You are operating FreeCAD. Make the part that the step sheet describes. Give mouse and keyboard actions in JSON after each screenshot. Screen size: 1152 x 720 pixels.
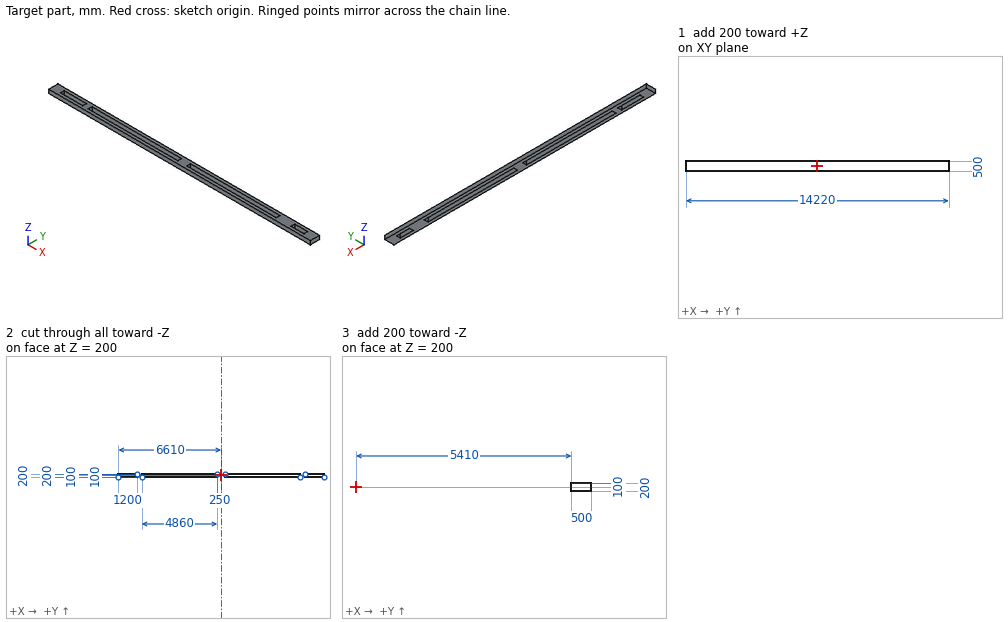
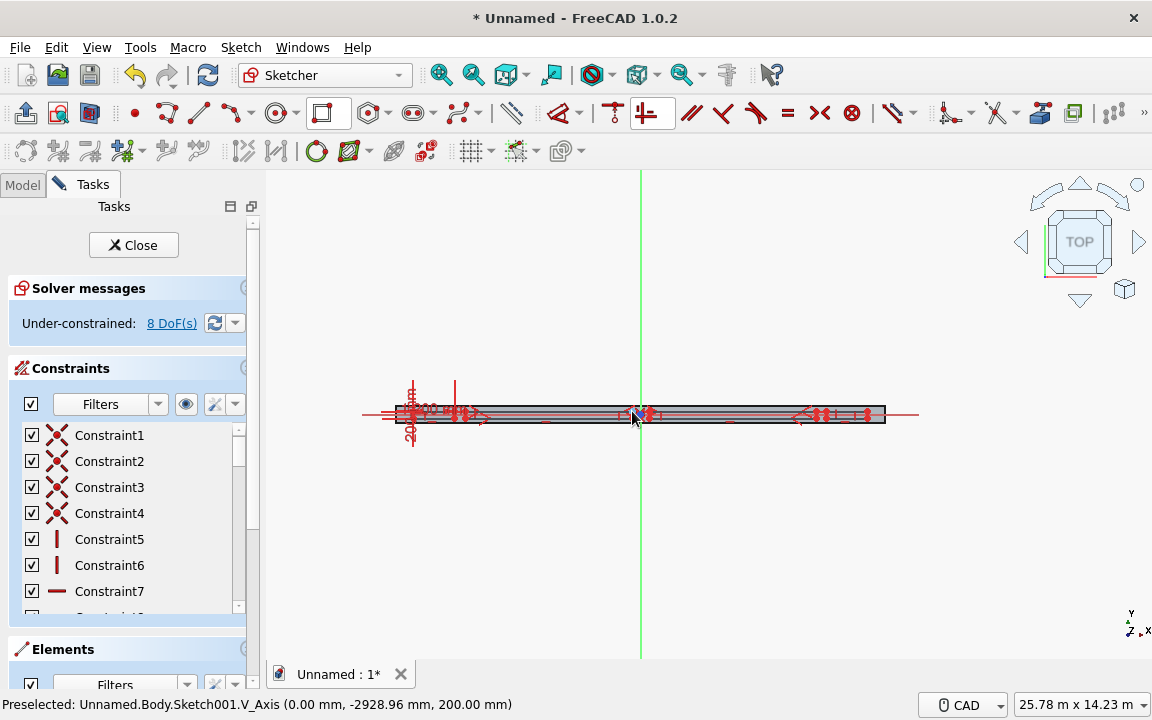
{"action": "scroll", "coordinate": [413, 419], "scroll_direction": "up", "scroll_amount": 3}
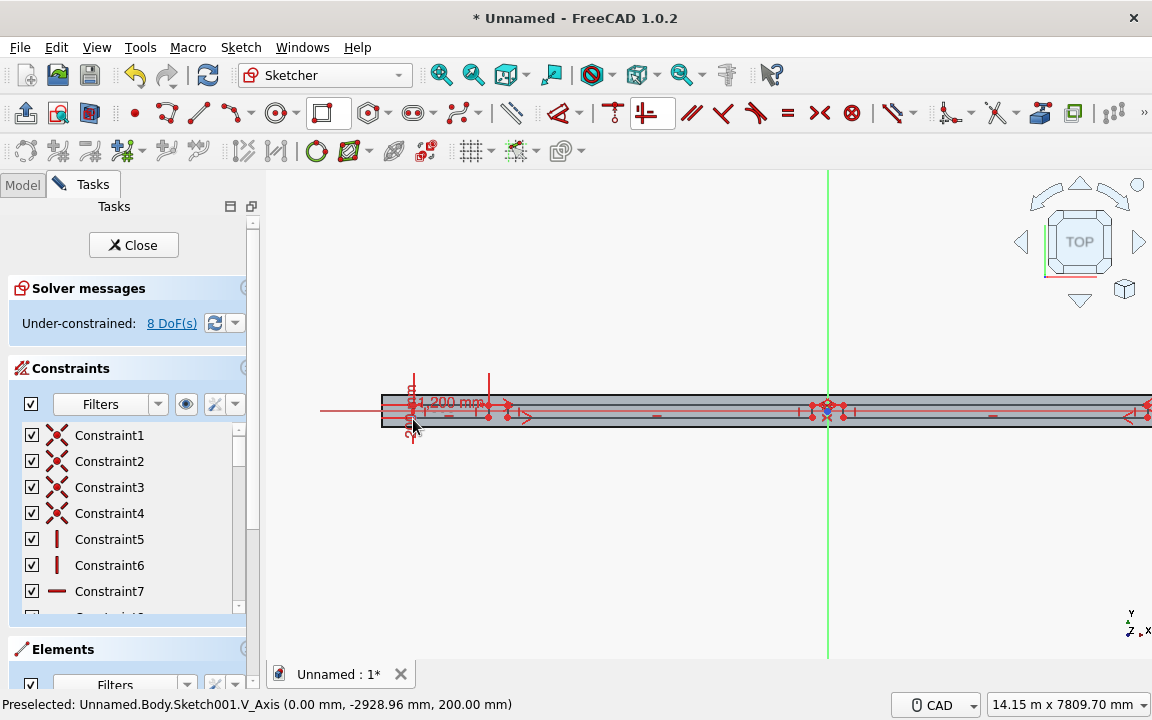
{"action": "left_click", "coordinate": [414, 418]}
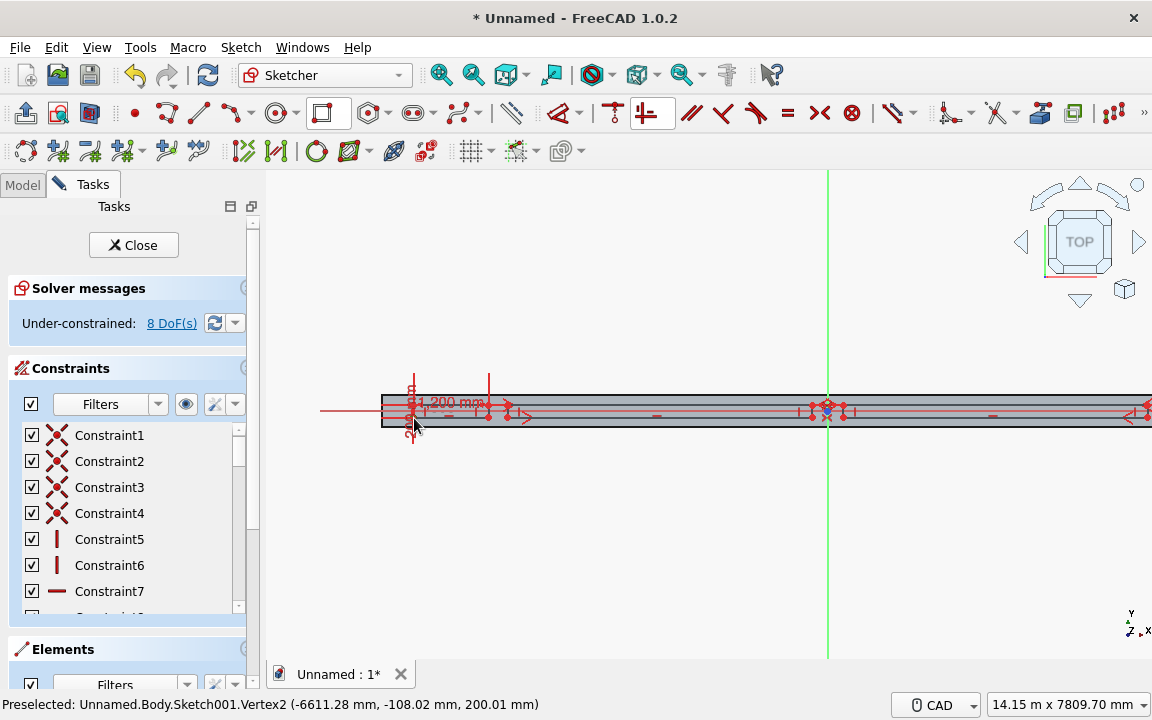
{"action": "scroll", "coordinate": [413, 419], "scroll_direction": "down", "scroll_amount": 3}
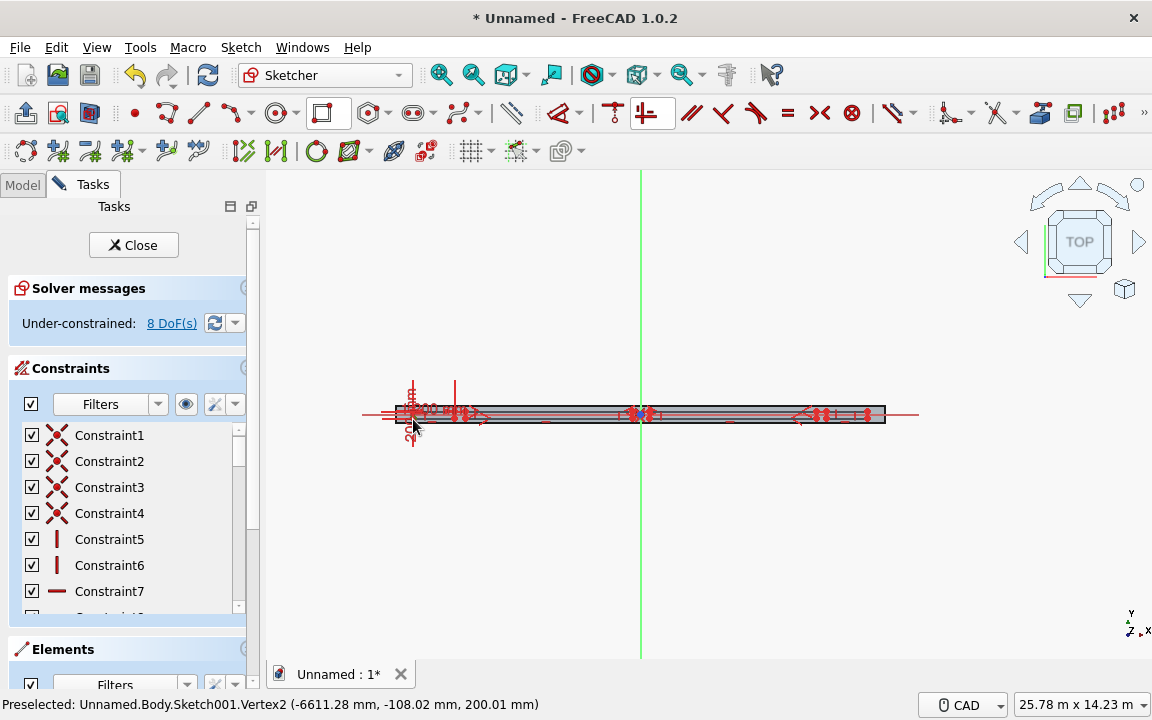
{"action": "scroll", "coordinate": [868, 419], "scroll_direction": "up", "scroll_amount": 3}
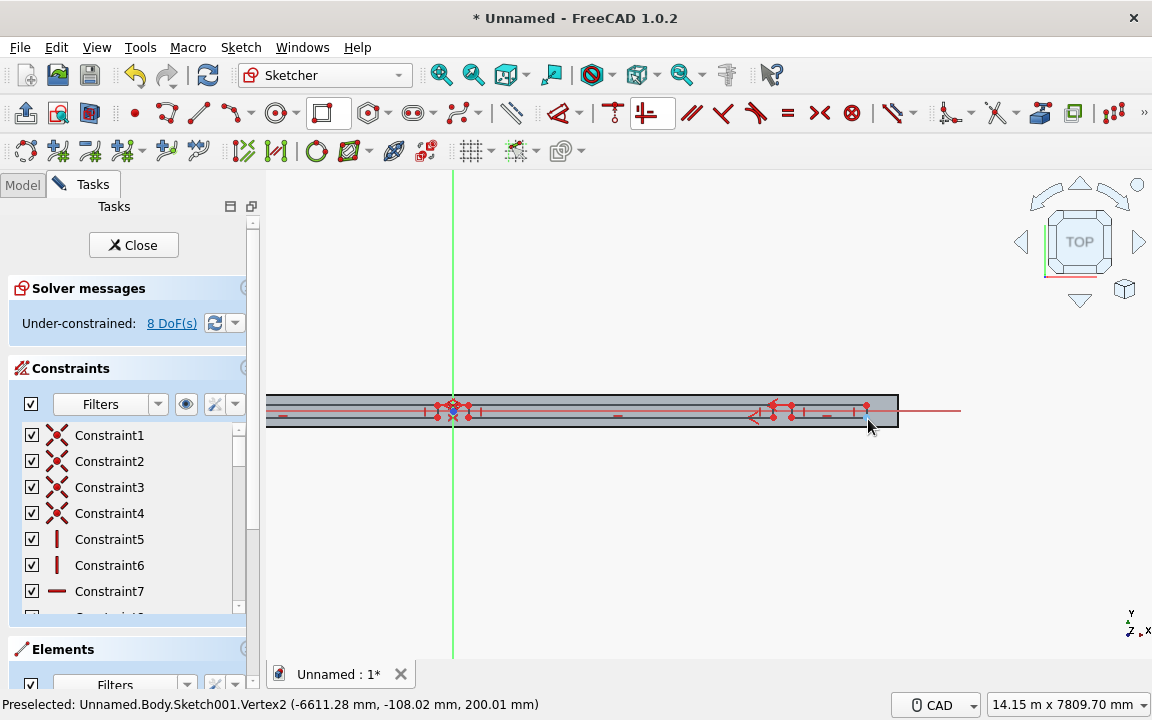
{"action": "left_click", "coordinate": [867, 418]}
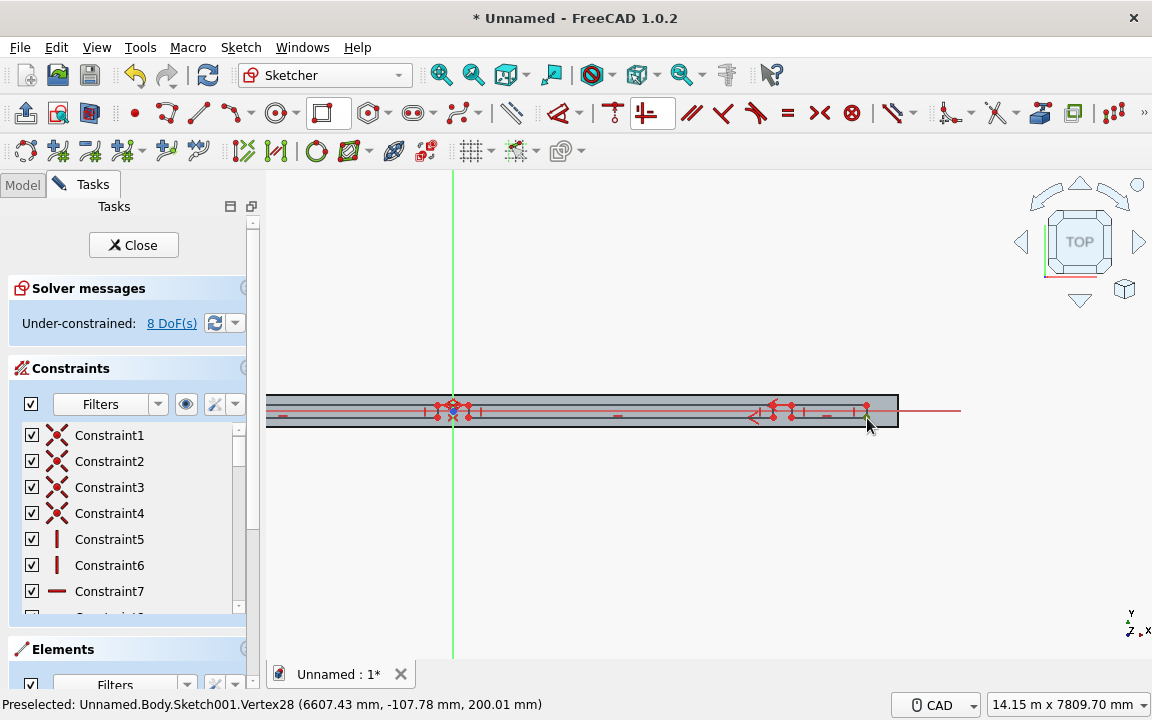
{"action": "left_click", "coordinate": [453, 600]}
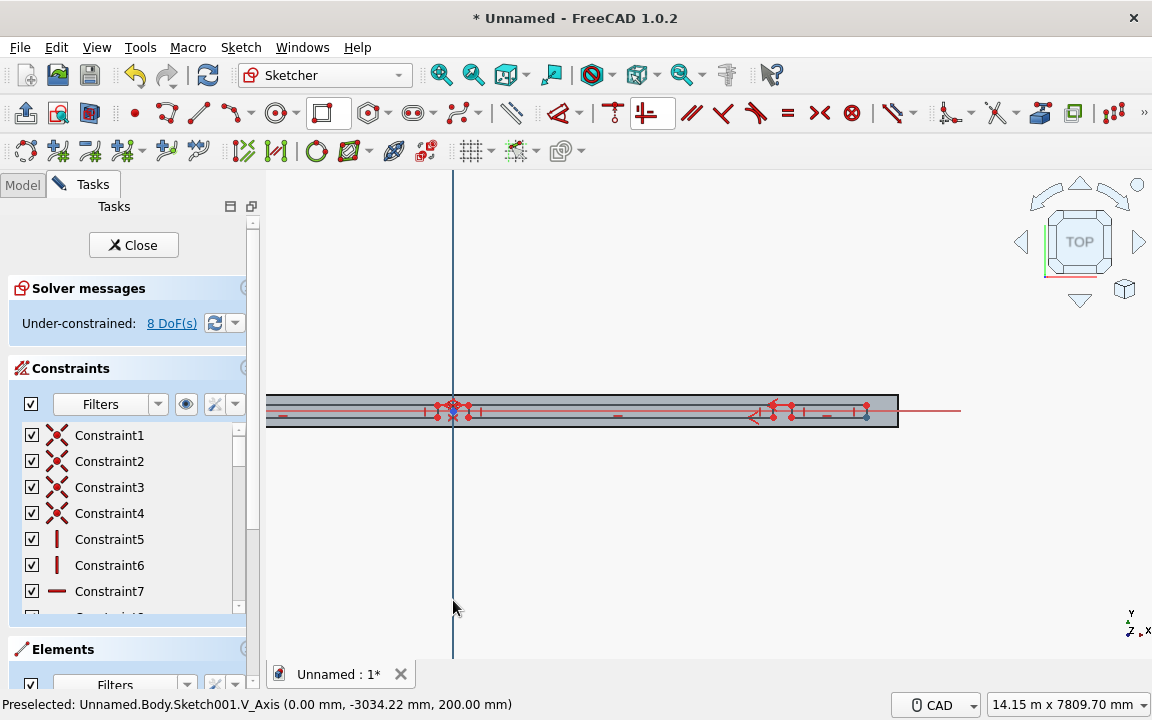
{"action": "left_click", "coordinate": [820, 114]}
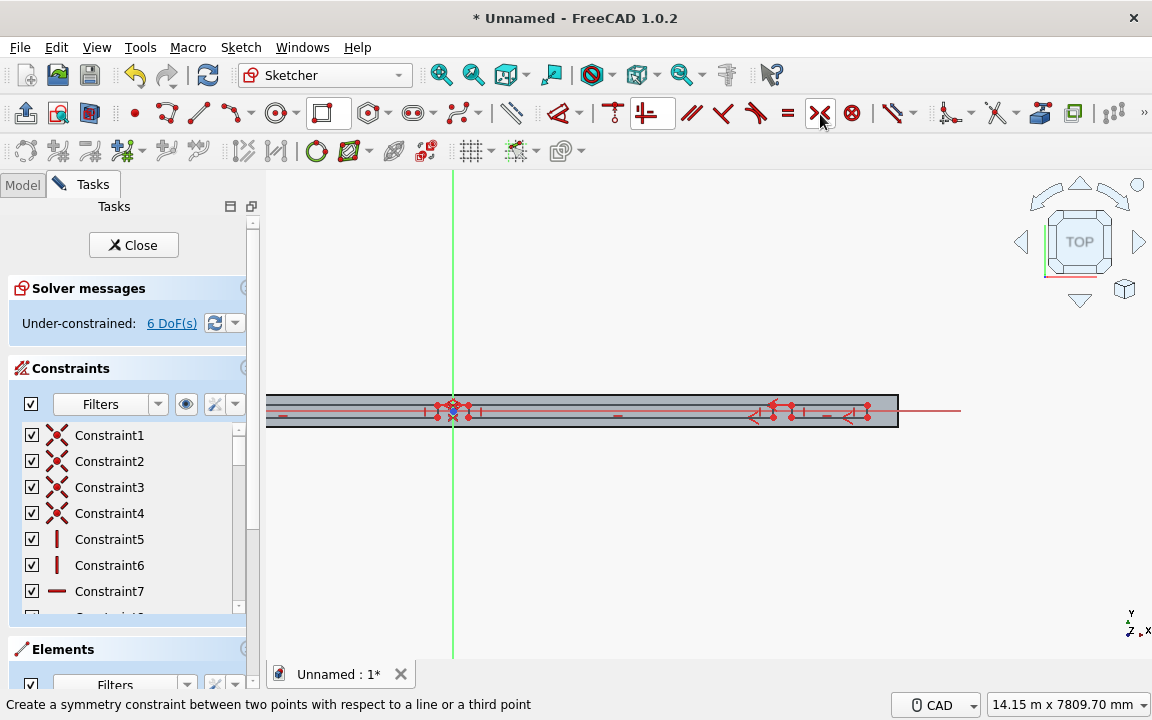
{"action": "left_click", "coordinate": [558, 114]}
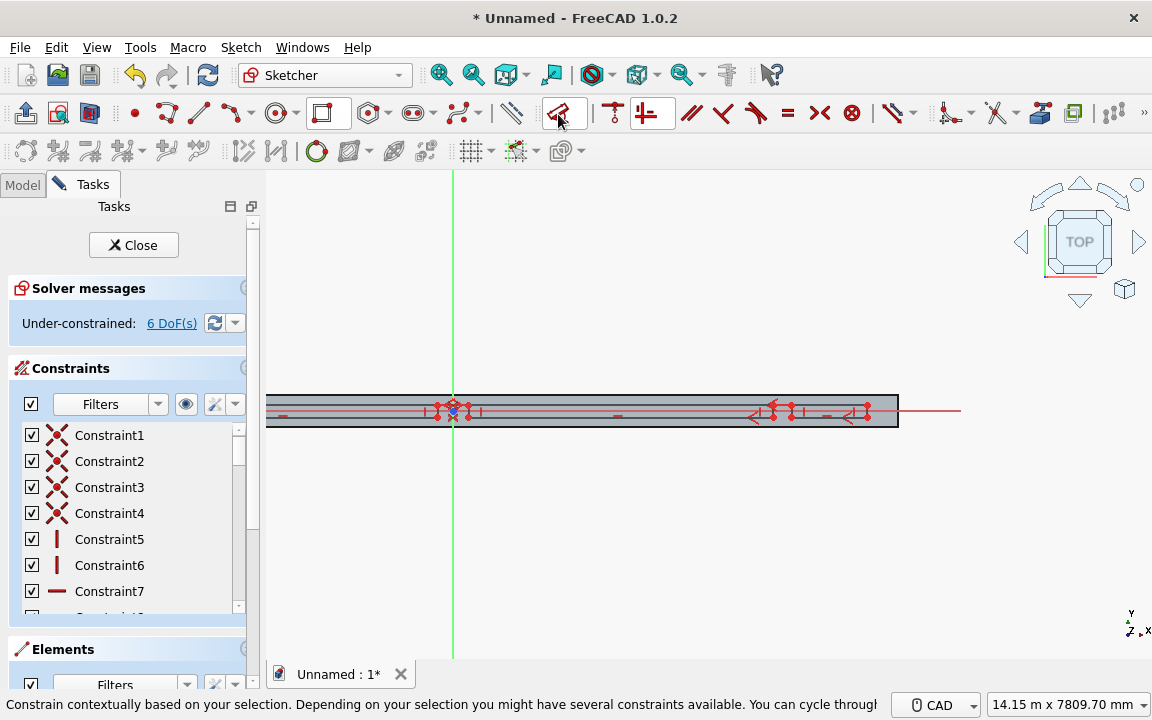
{"action": "scroll", "coordinate": [868, 419], "scroll_direction": "down", "scroll_amount": 3}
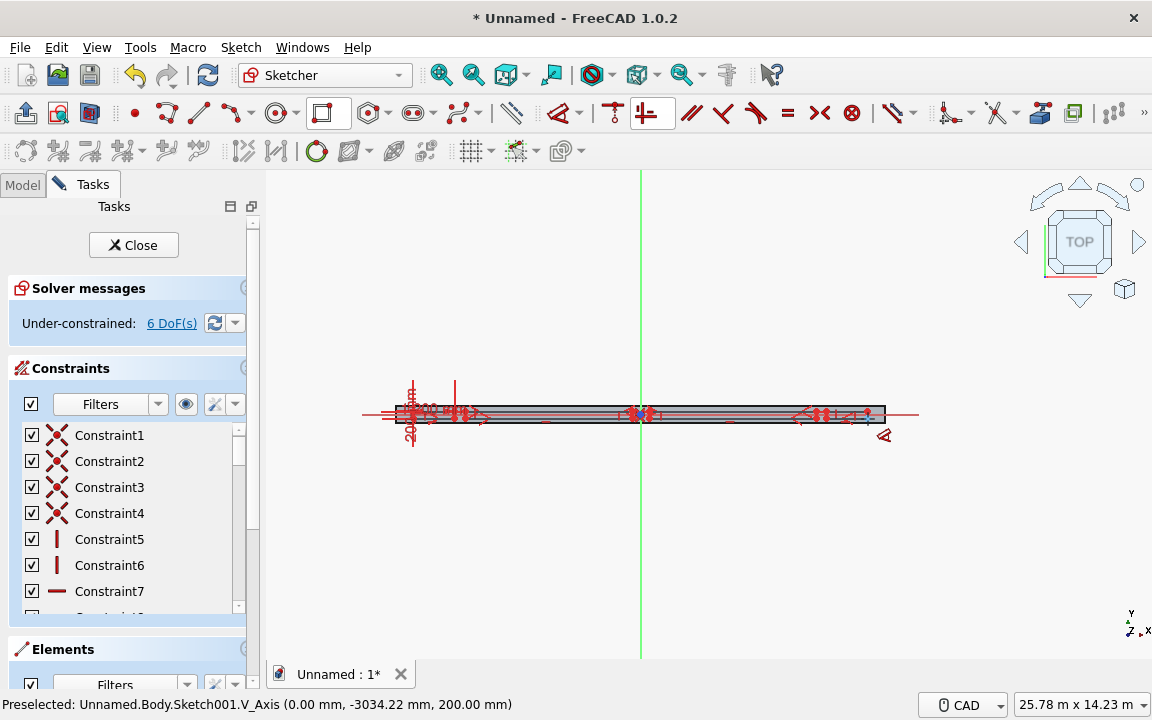
{"action": "scroll", "coordinate": [465, 415], "scroll_direction": "up", "scroll_amount": 9}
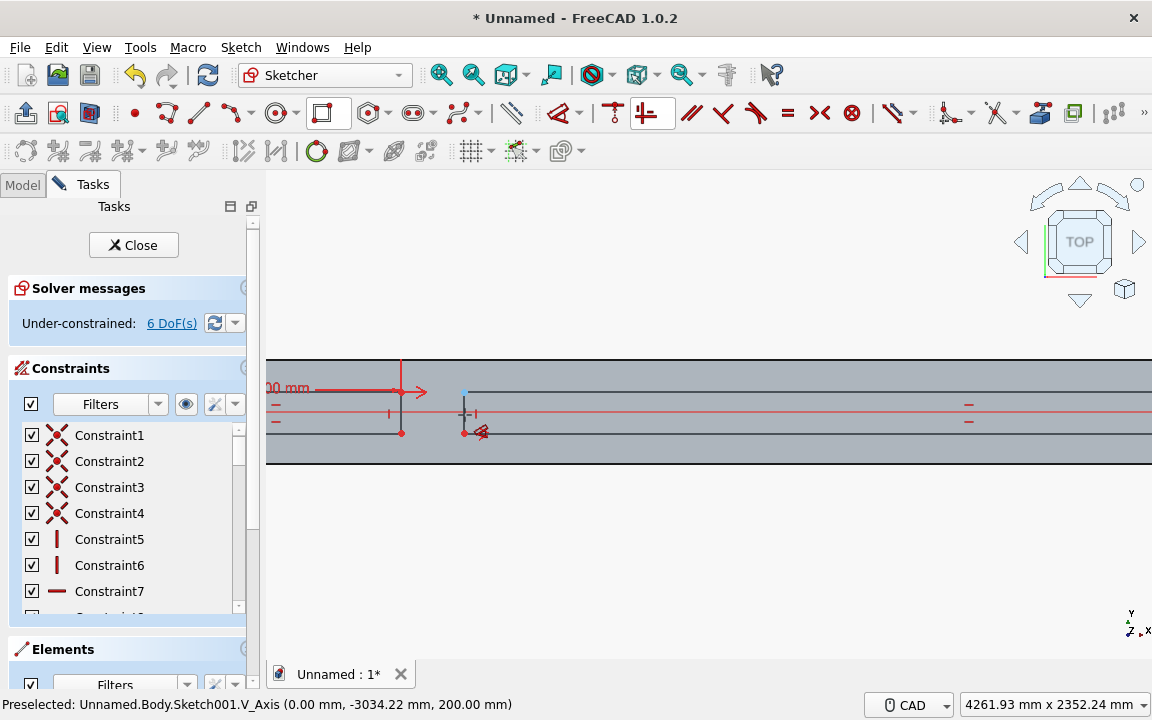
{"action": "left_click", "coordinate": [464, 413]}
{"action": "left_click", "coordinate": [430, 398]}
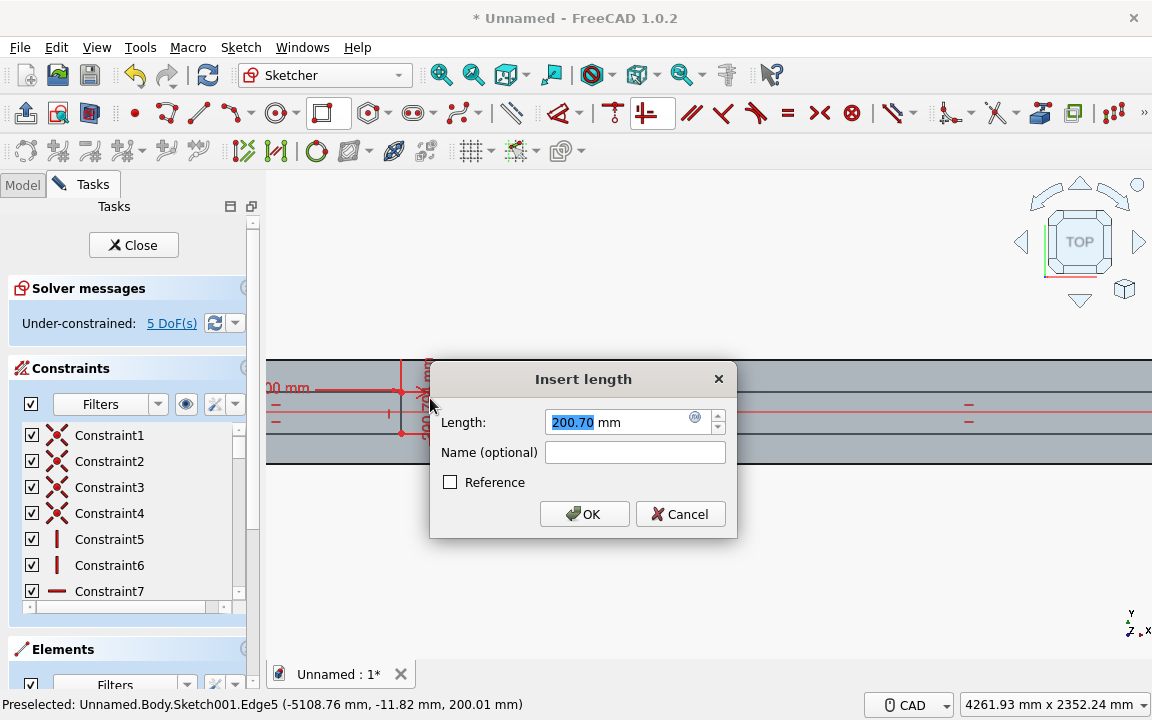
{"action": "type", "text": "200"}
{"action": "key", "text": "Return"}